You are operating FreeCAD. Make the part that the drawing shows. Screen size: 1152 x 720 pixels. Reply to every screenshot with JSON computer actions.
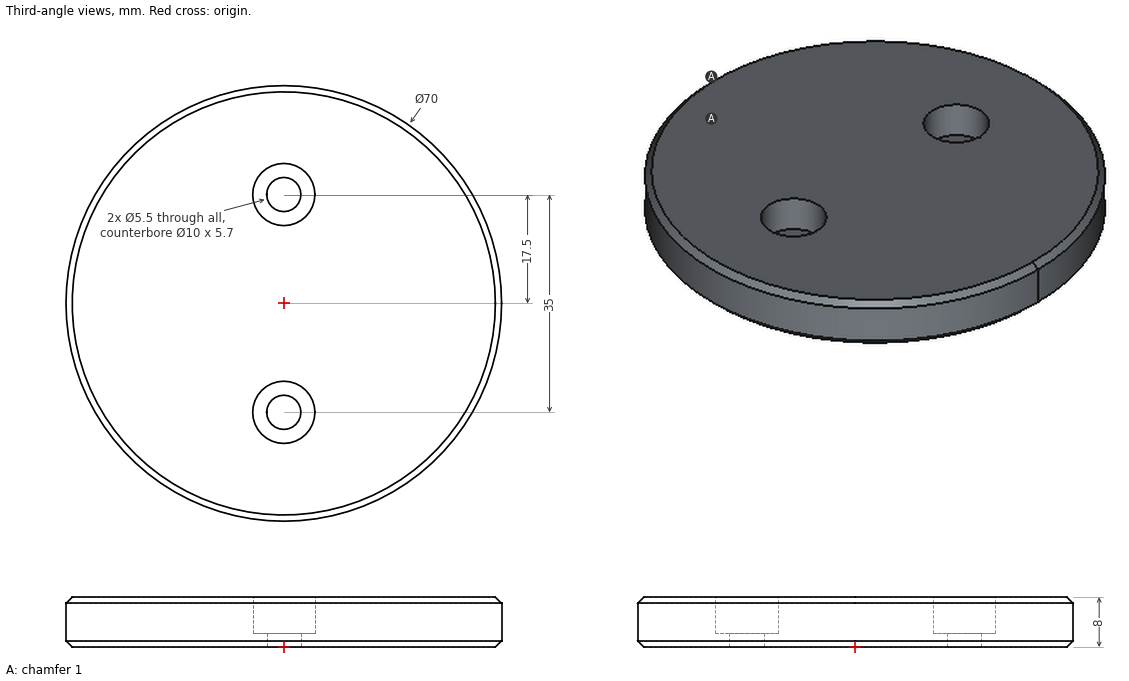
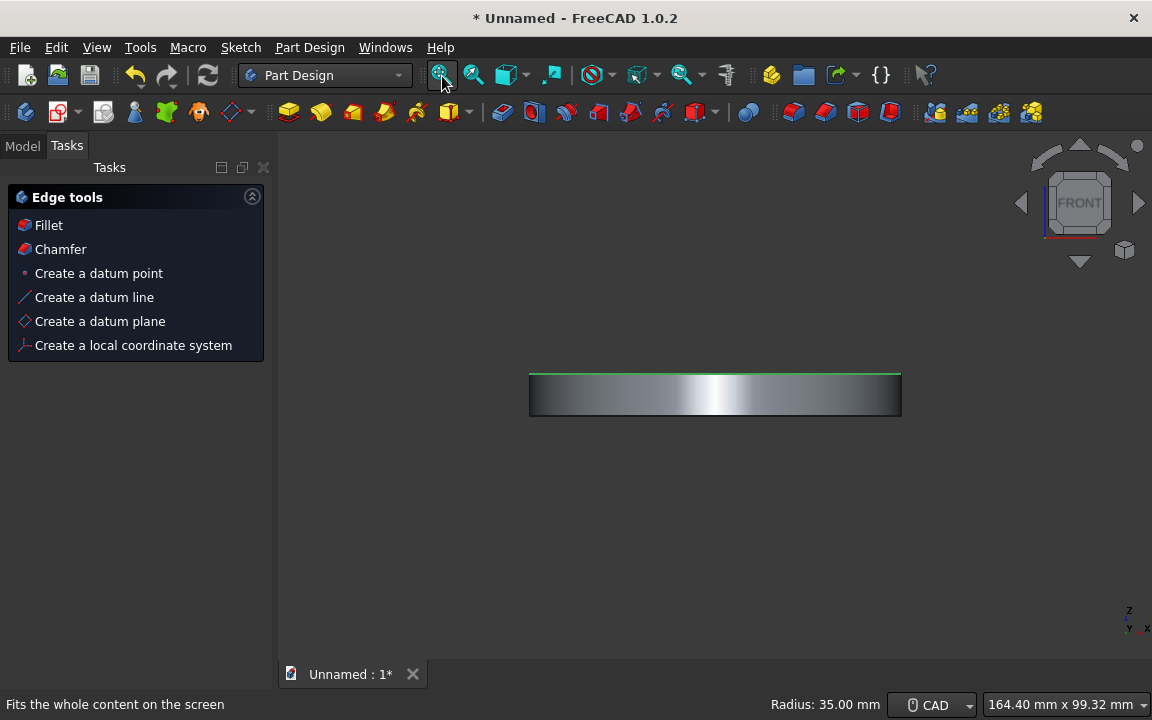
{"action": "left_click", "coordinate": [564, 415], "text": "ctrl"}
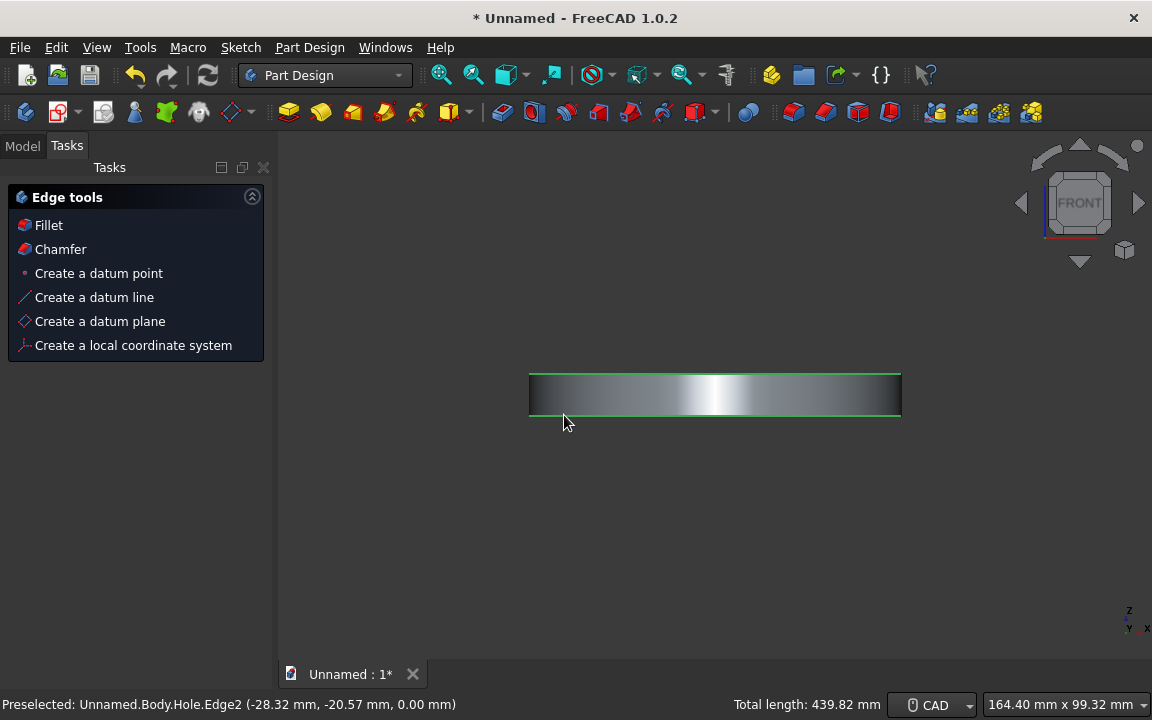
{"action": "left_click", "coordinate": [826, 112]}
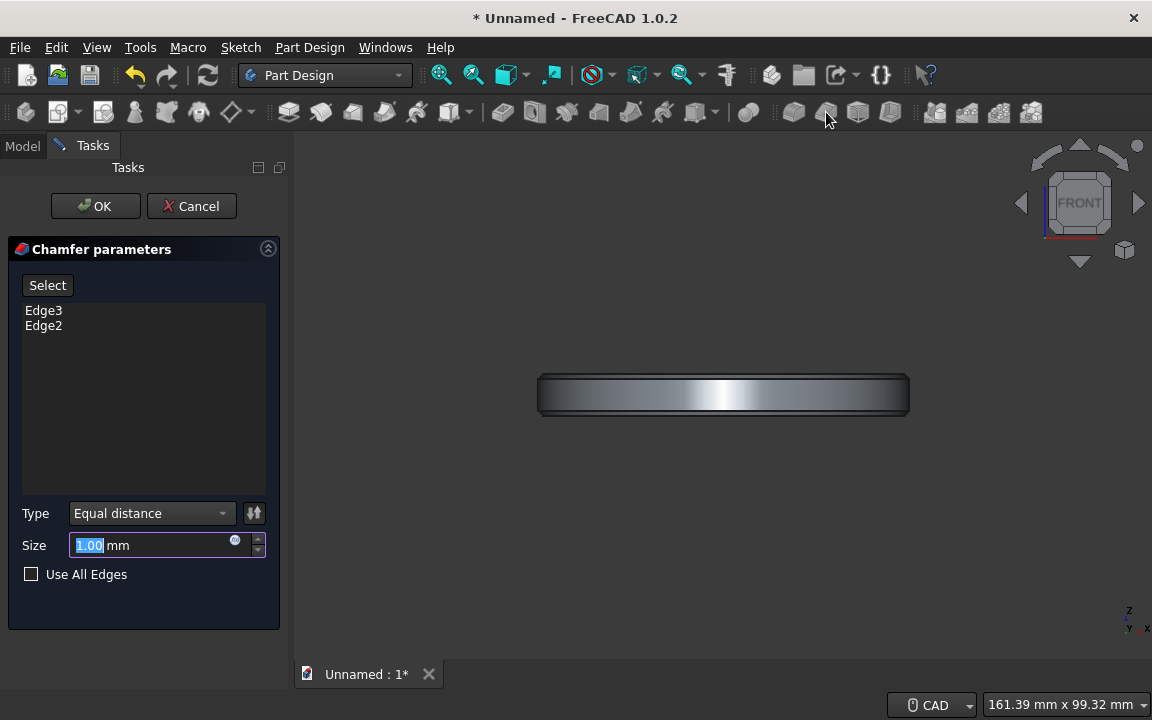
{"action": "type", "text": "1"}
{"action": "key", "text": "Tab"}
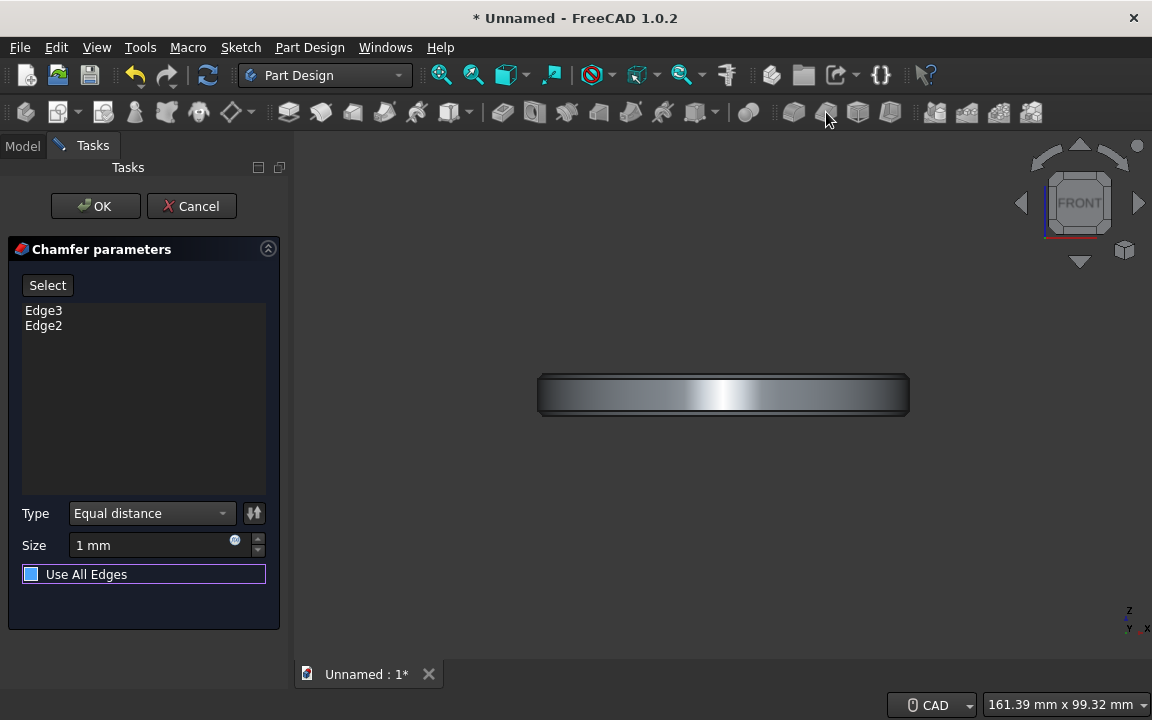
{"action": "left_click", "coordinate": [96, 206]}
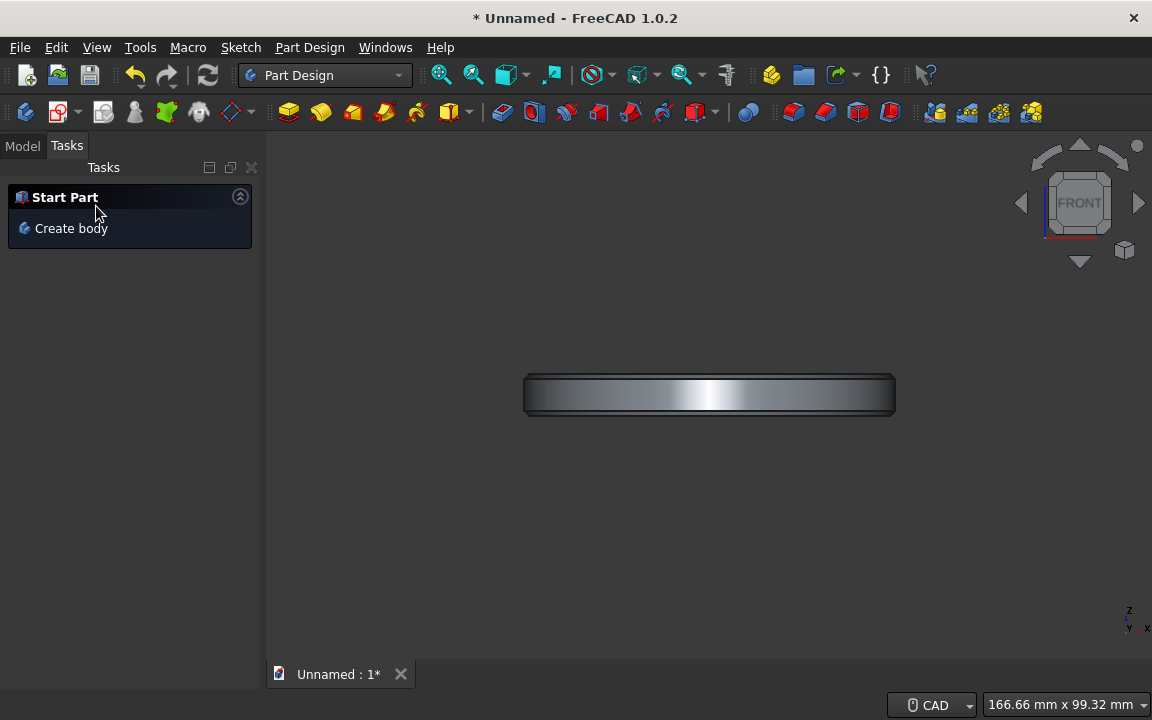
{"action": "key", "text": "0"}